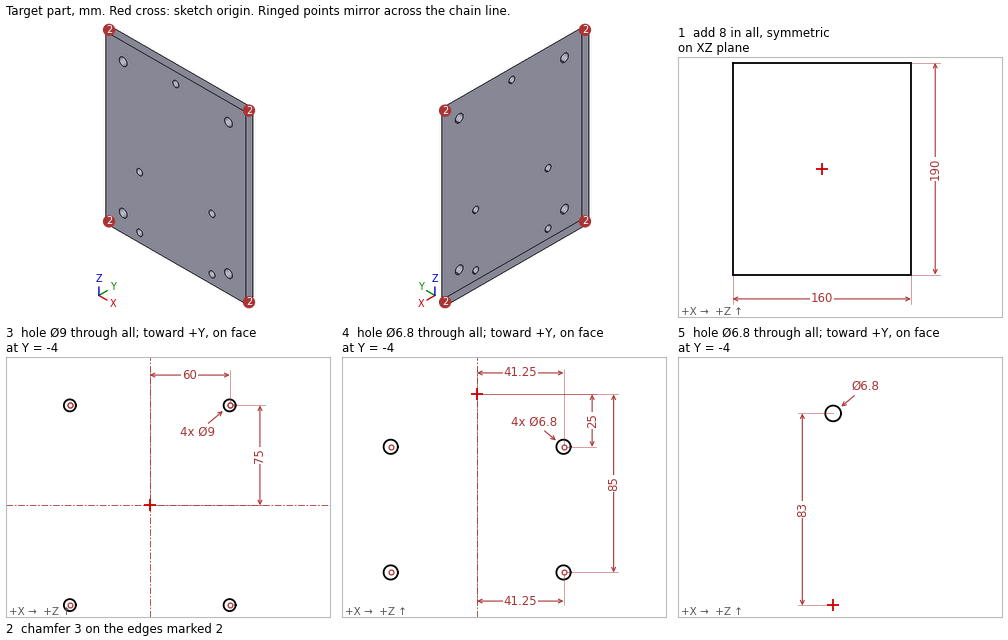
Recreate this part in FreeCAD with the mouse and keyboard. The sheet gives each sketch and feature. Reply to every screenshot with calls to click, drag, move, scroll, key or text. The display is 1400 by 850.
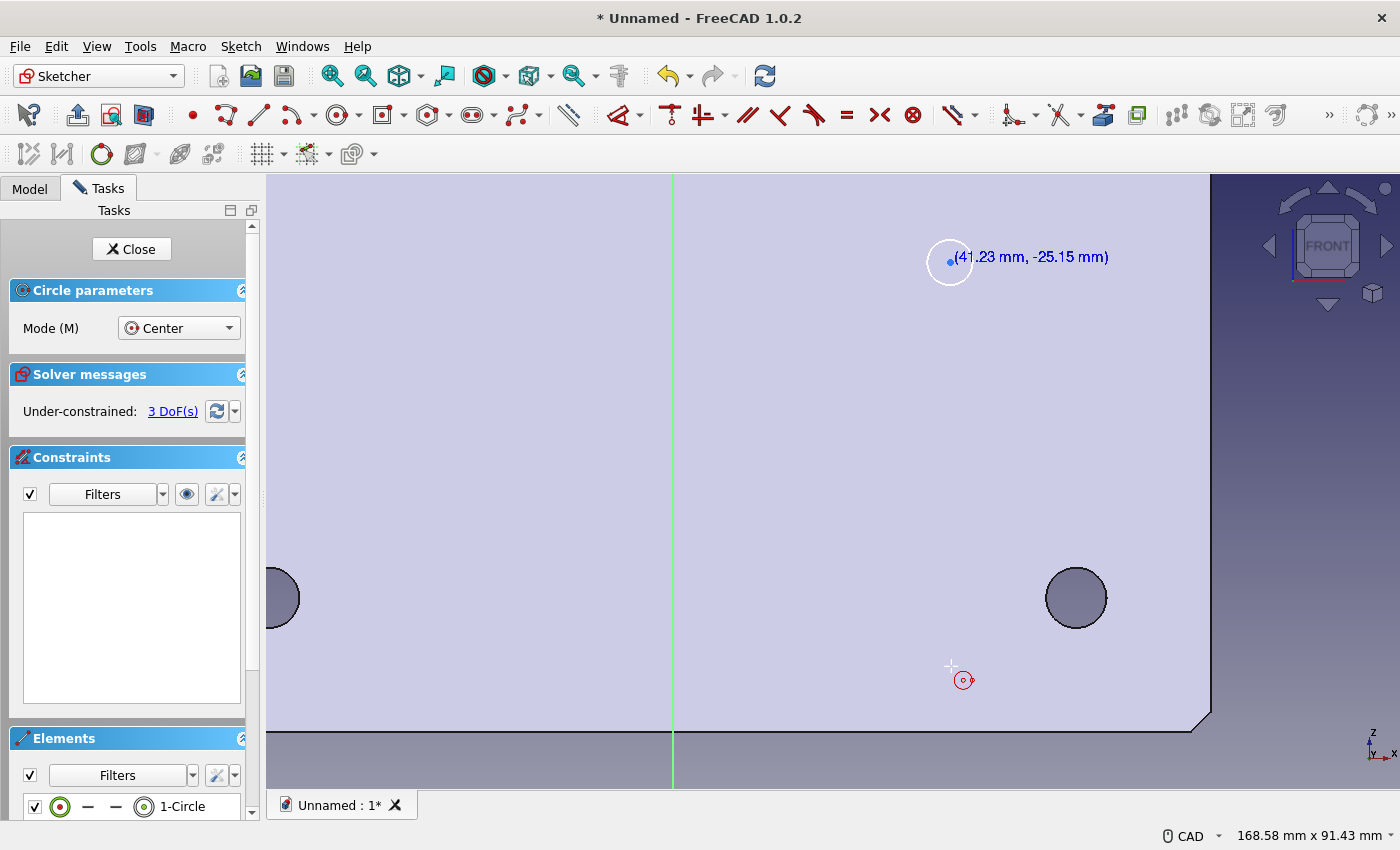
click(950, 665)
click(966, 649)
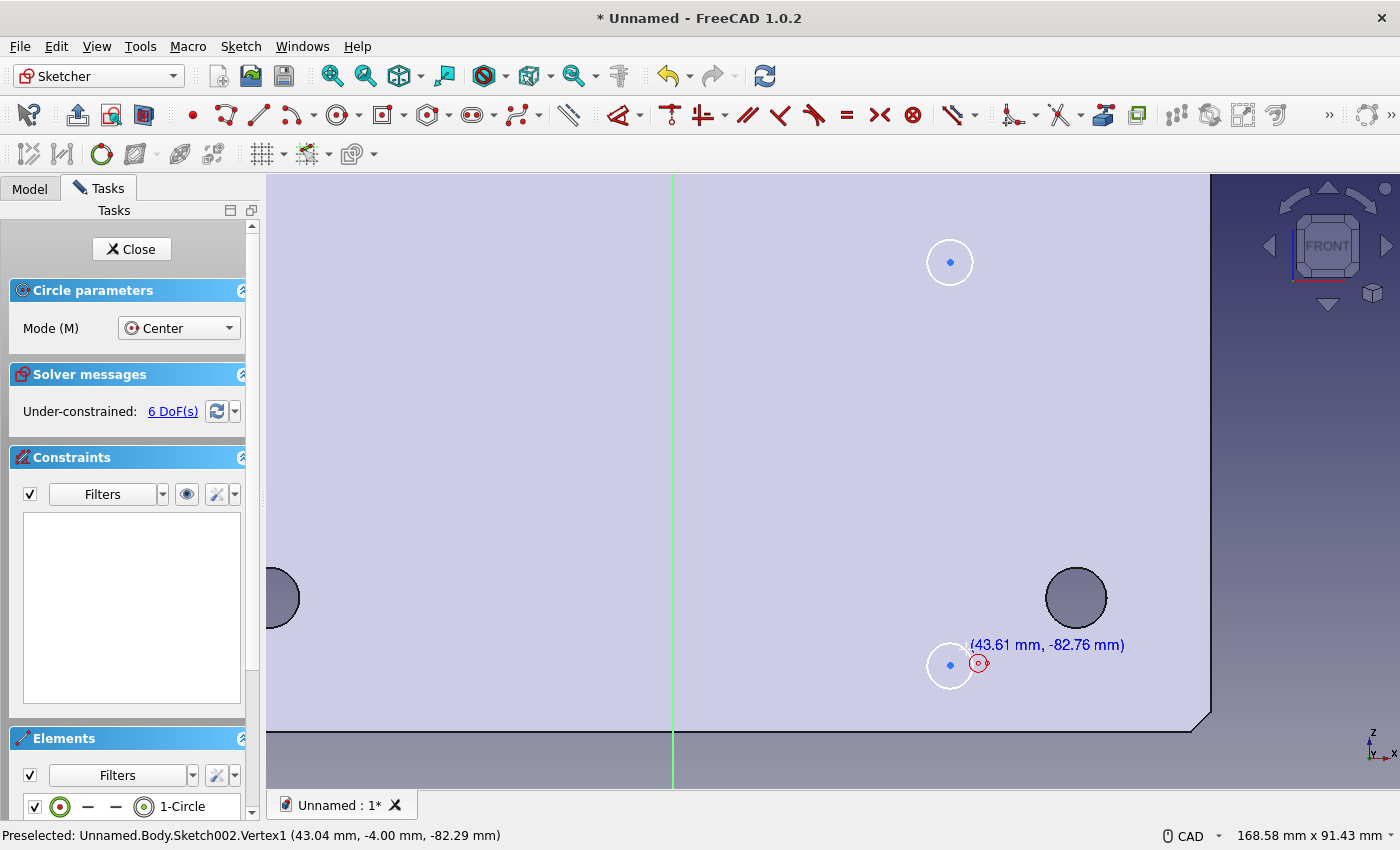
click(395, 665)
click(411, 649)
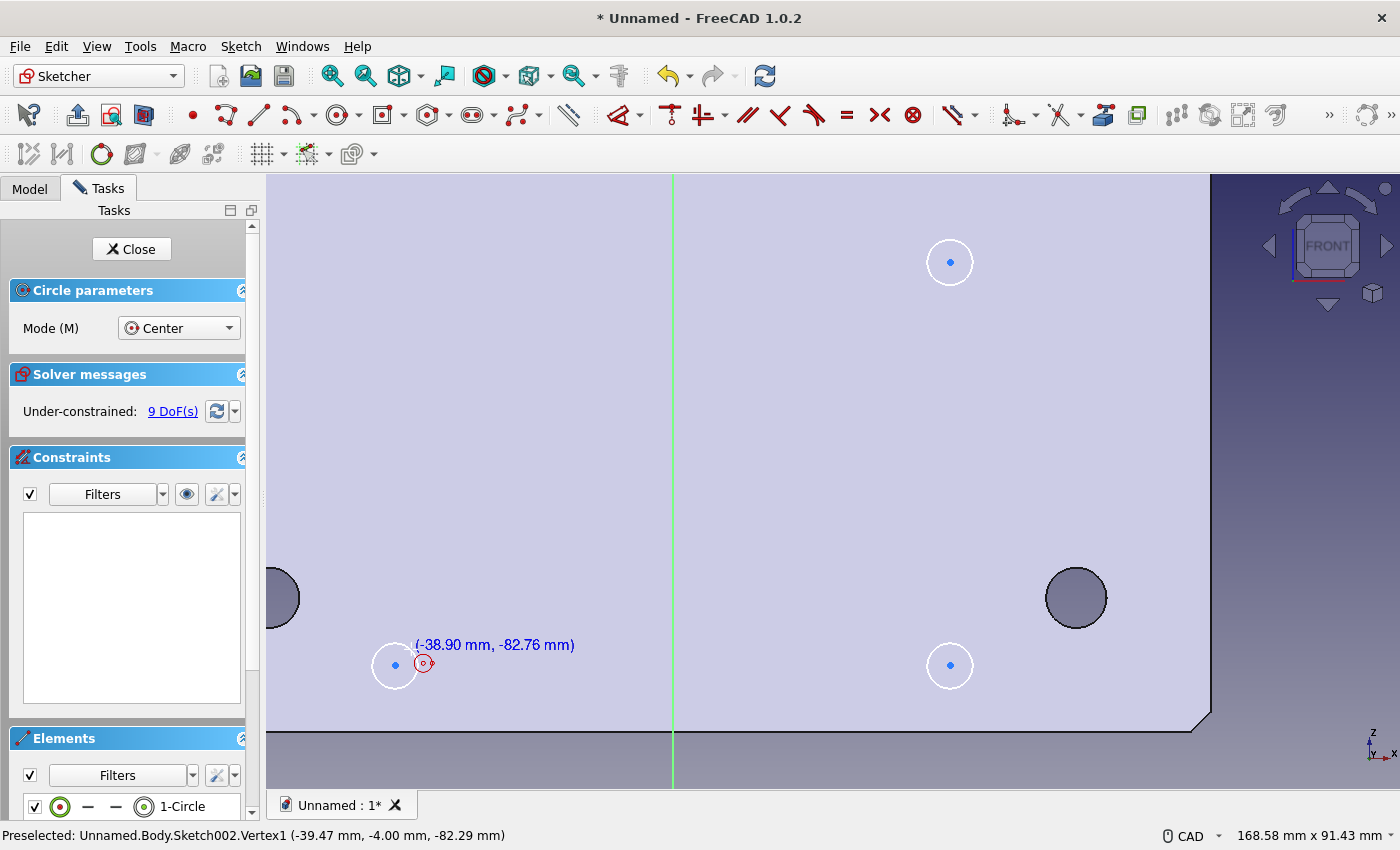
click(395, 261)
click(411, 245)
key(Escape)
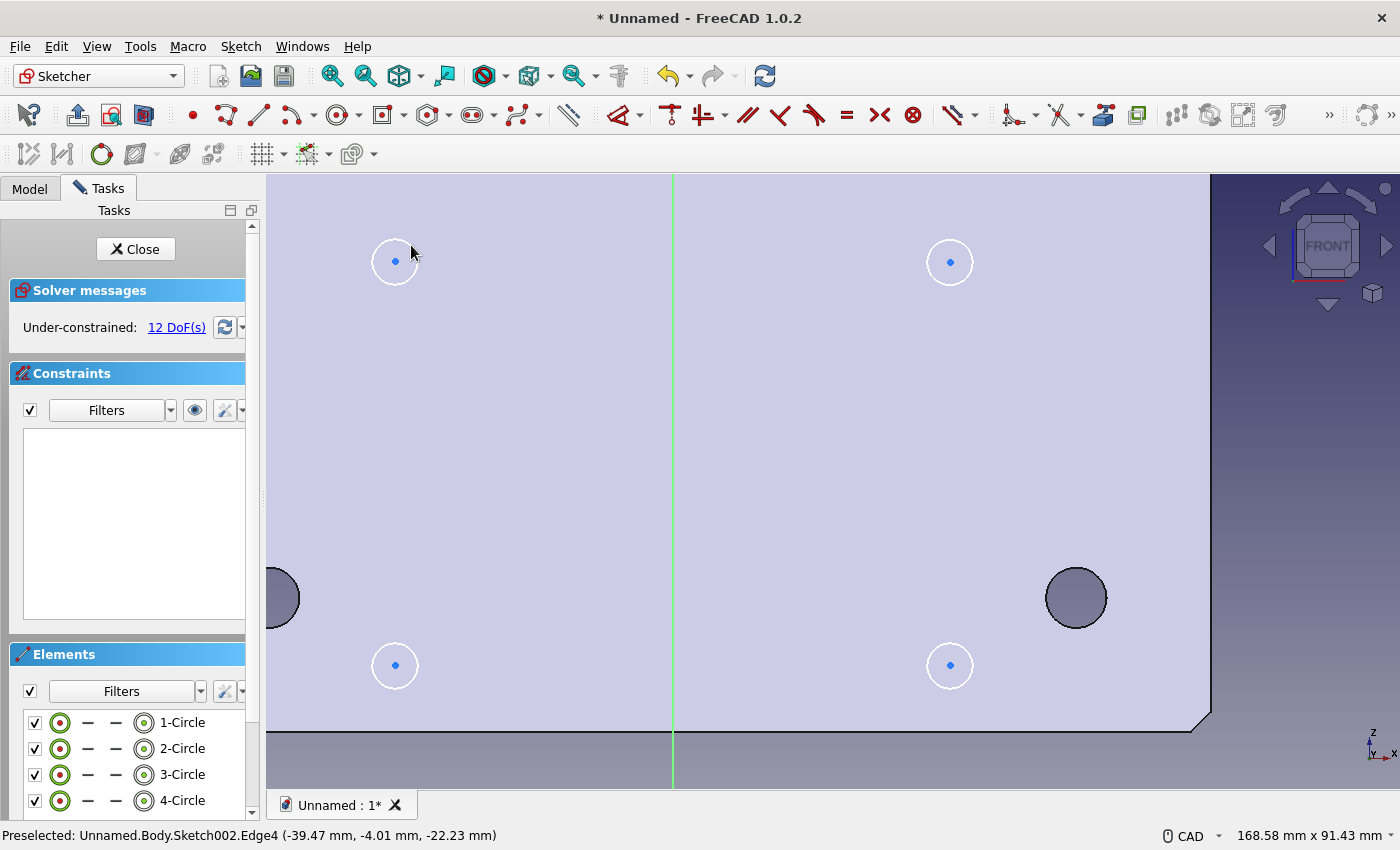
click(966, 246)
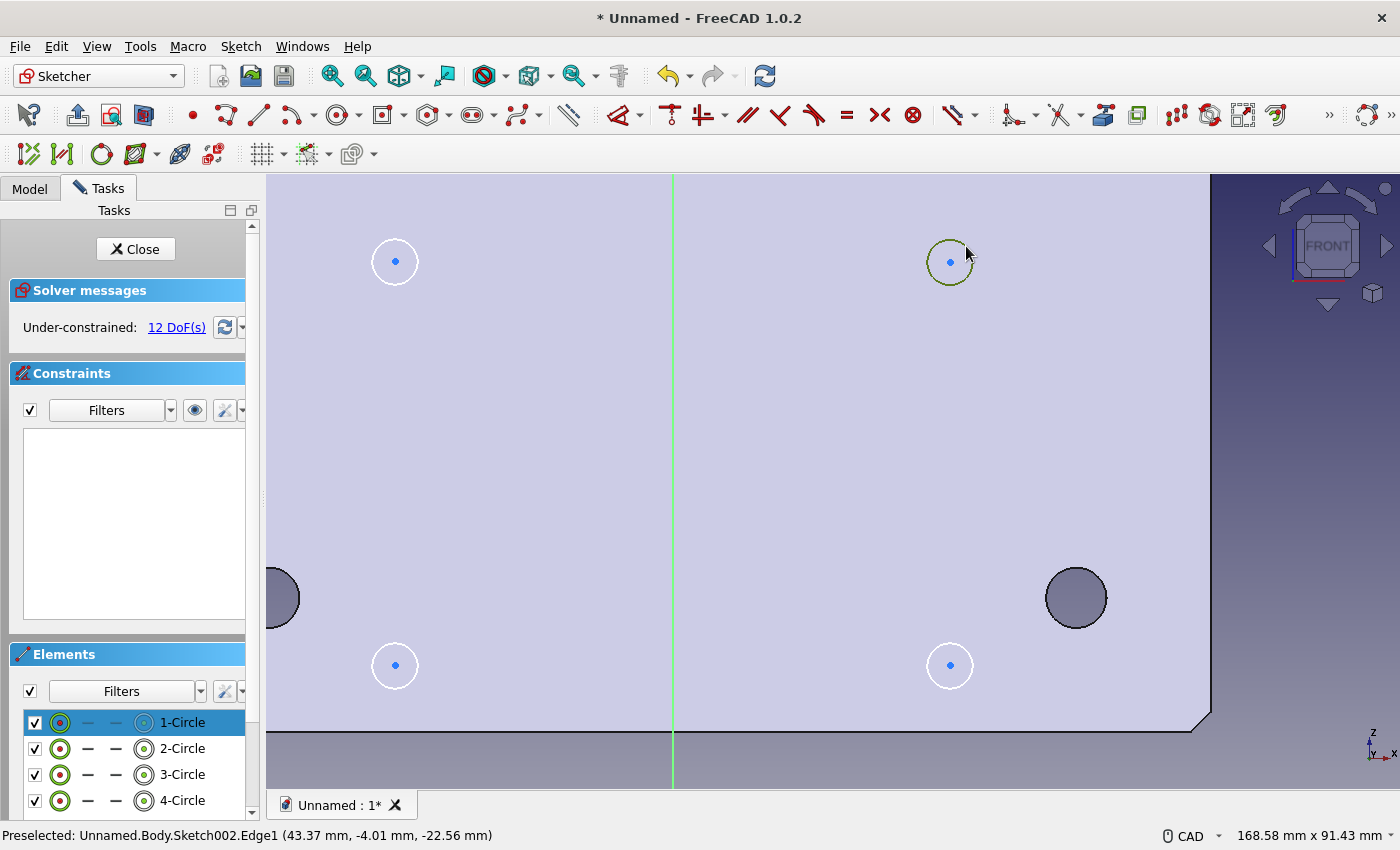
click(966, 650)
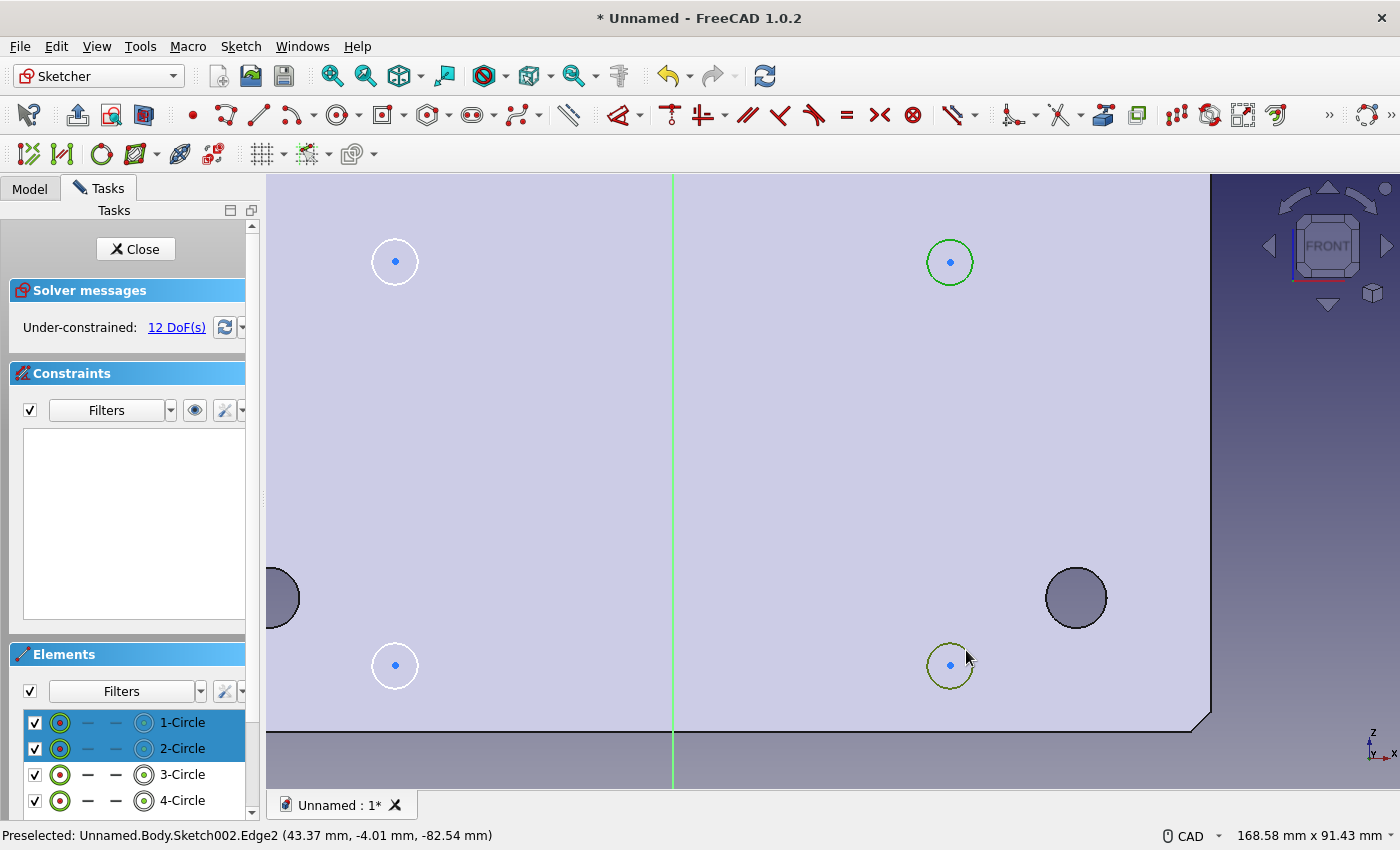
click(411, 650)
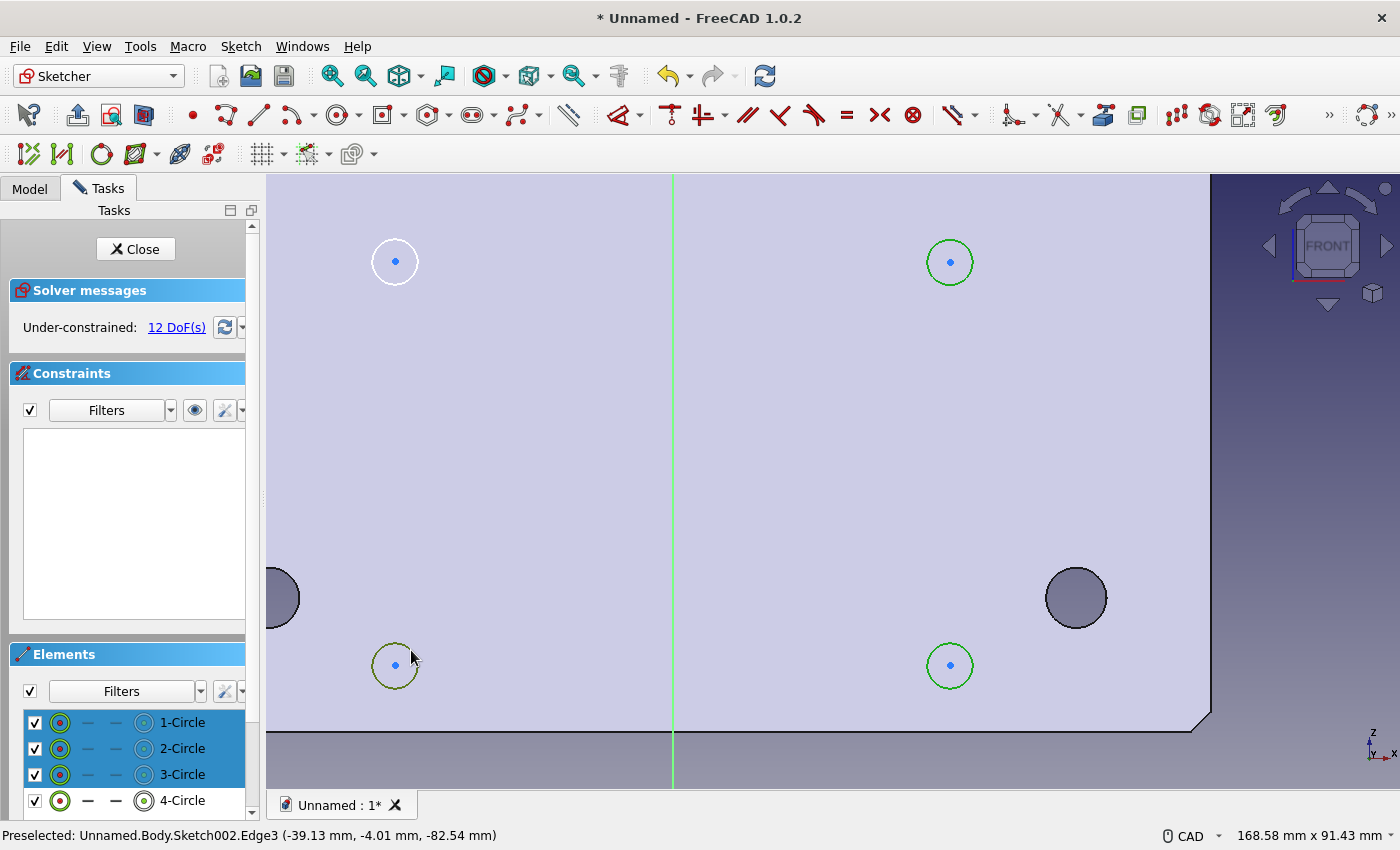
click(411, 246)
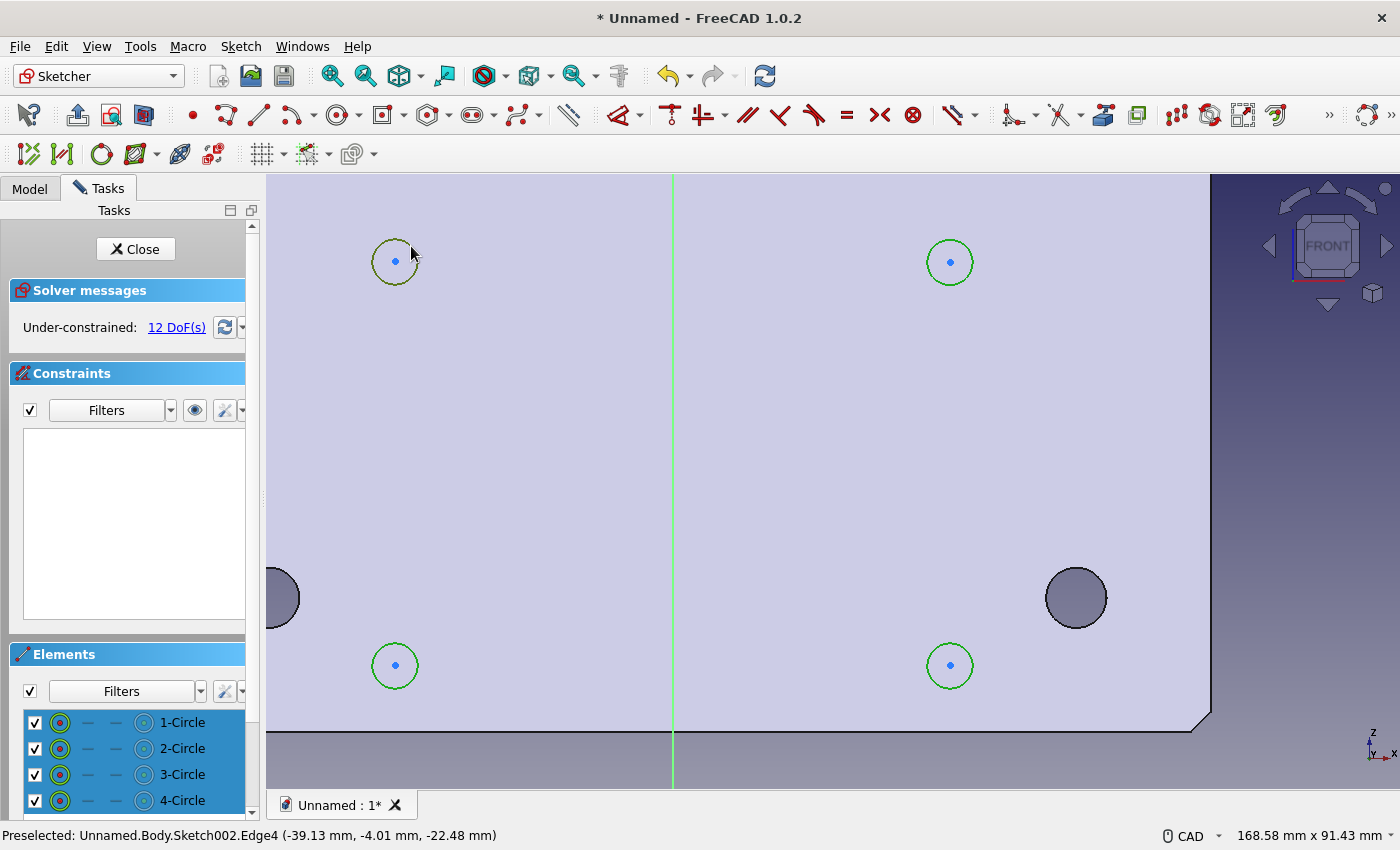
click(847, 116)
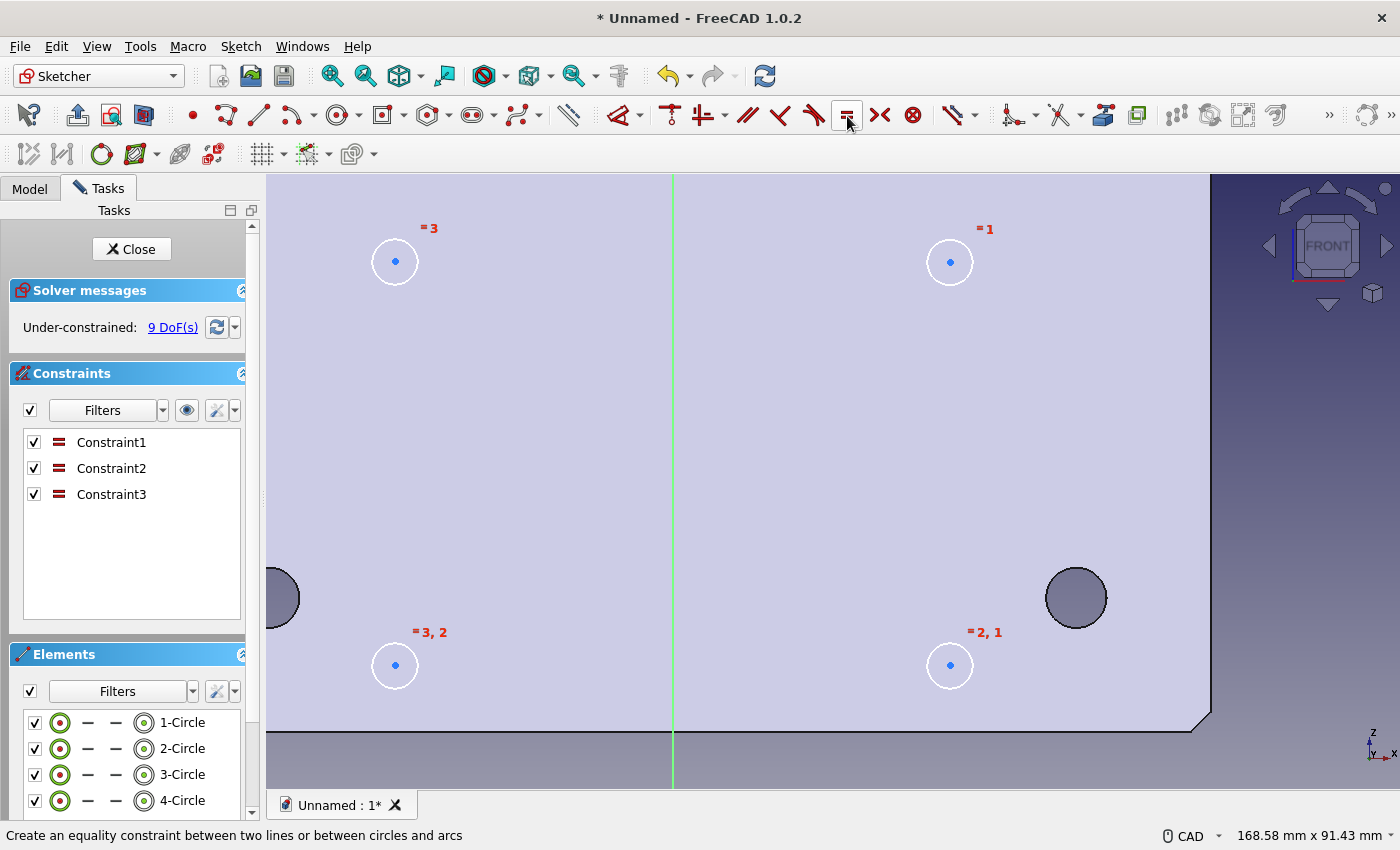
click(950, 666)